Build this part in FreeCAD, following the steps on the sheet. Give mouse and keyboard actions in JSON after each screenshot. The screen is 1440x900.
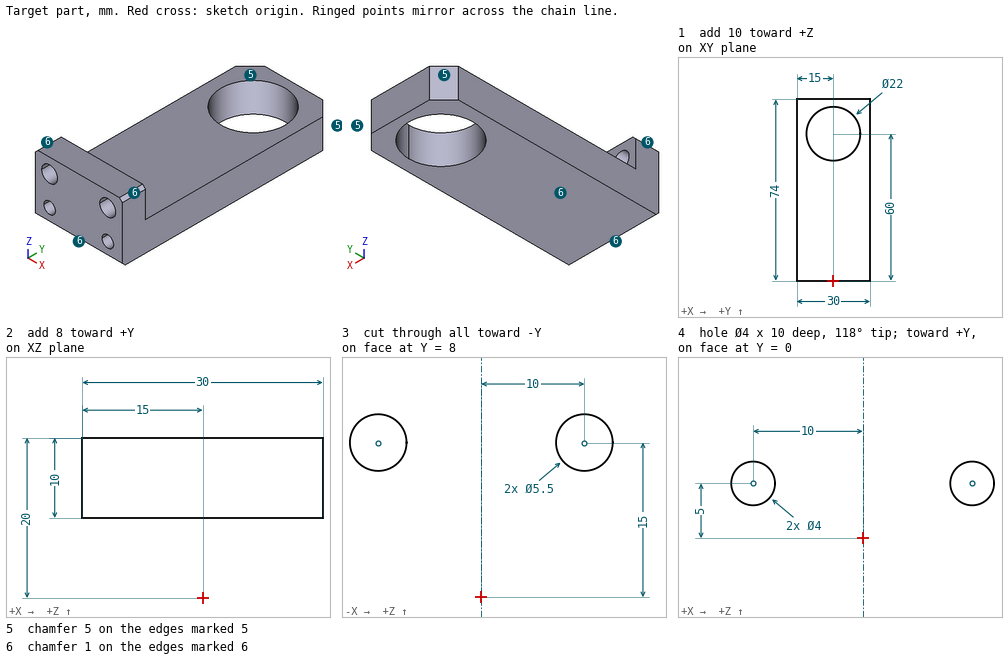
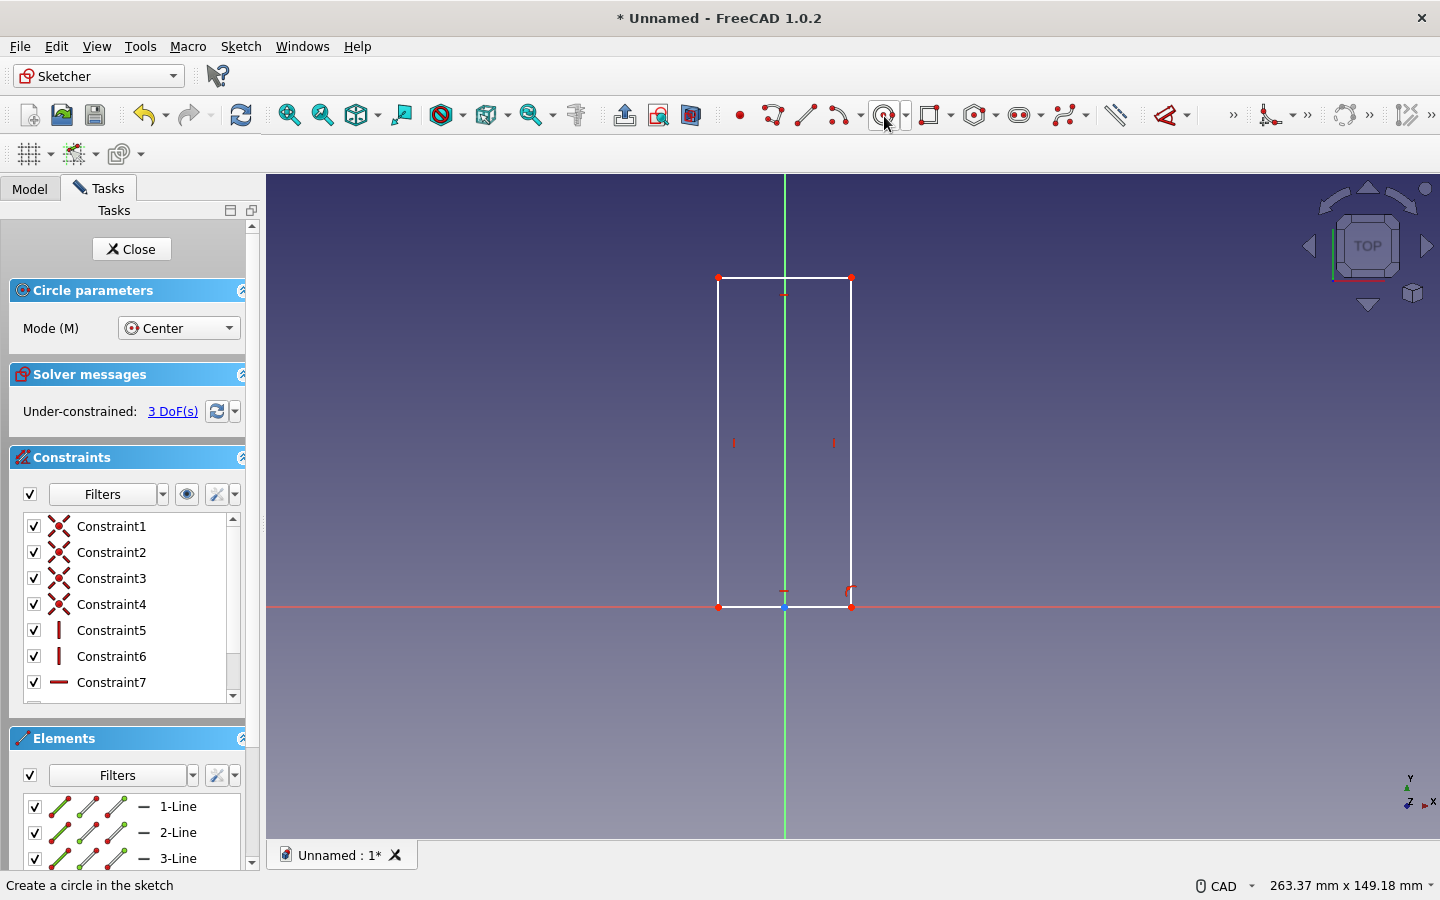
{"action": "left_click", "coordinate": [785, 340]}
{"action": "left_click", "coordinate": [819, 305]}
{"action": "key", "text": "Escape"}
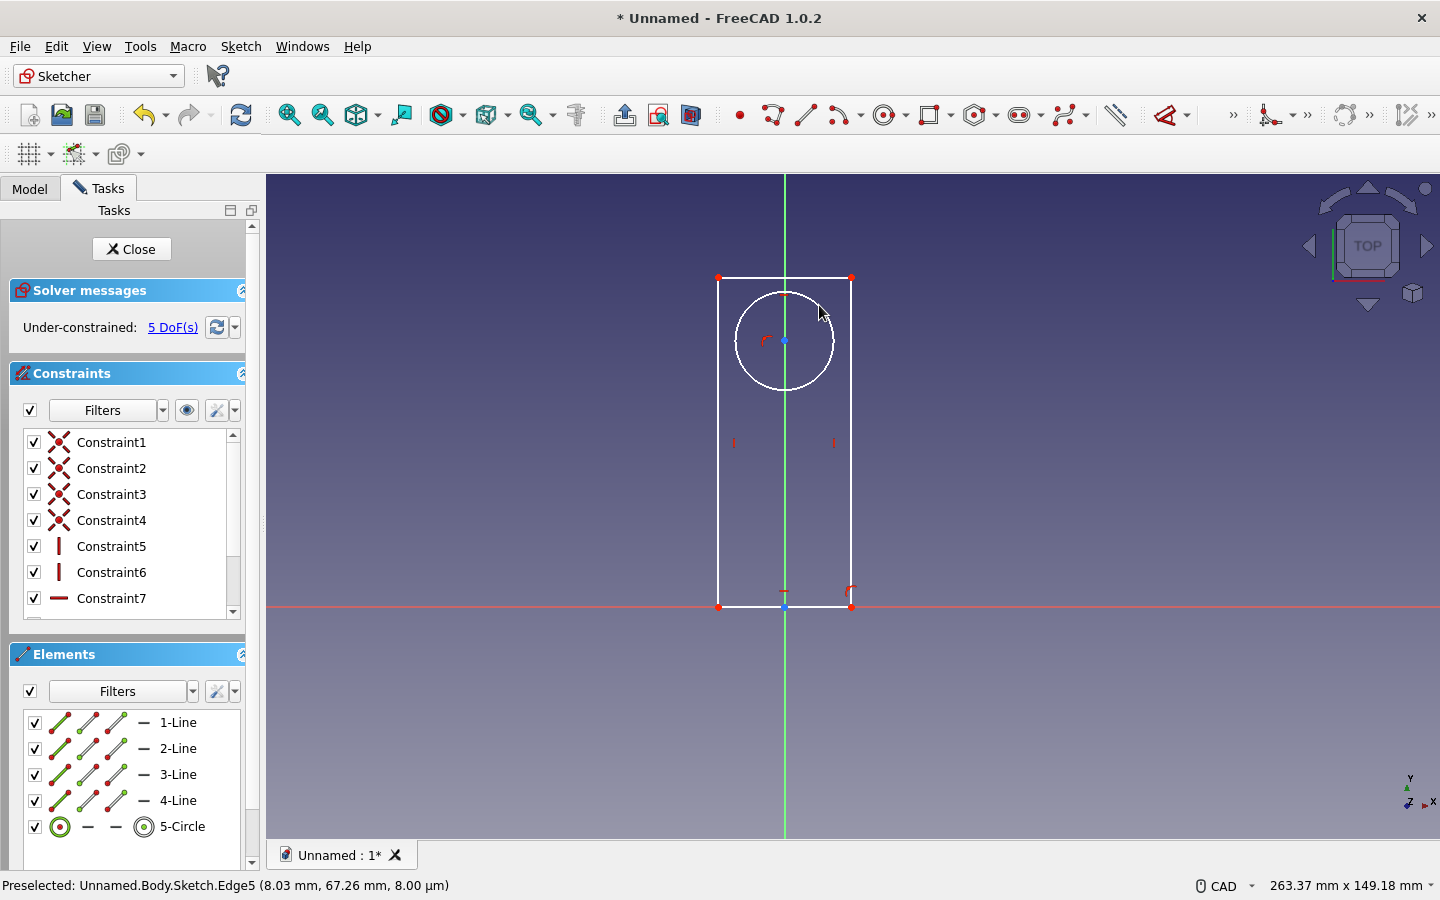
{"action": "left_click", "coordinate": [1164, 116]}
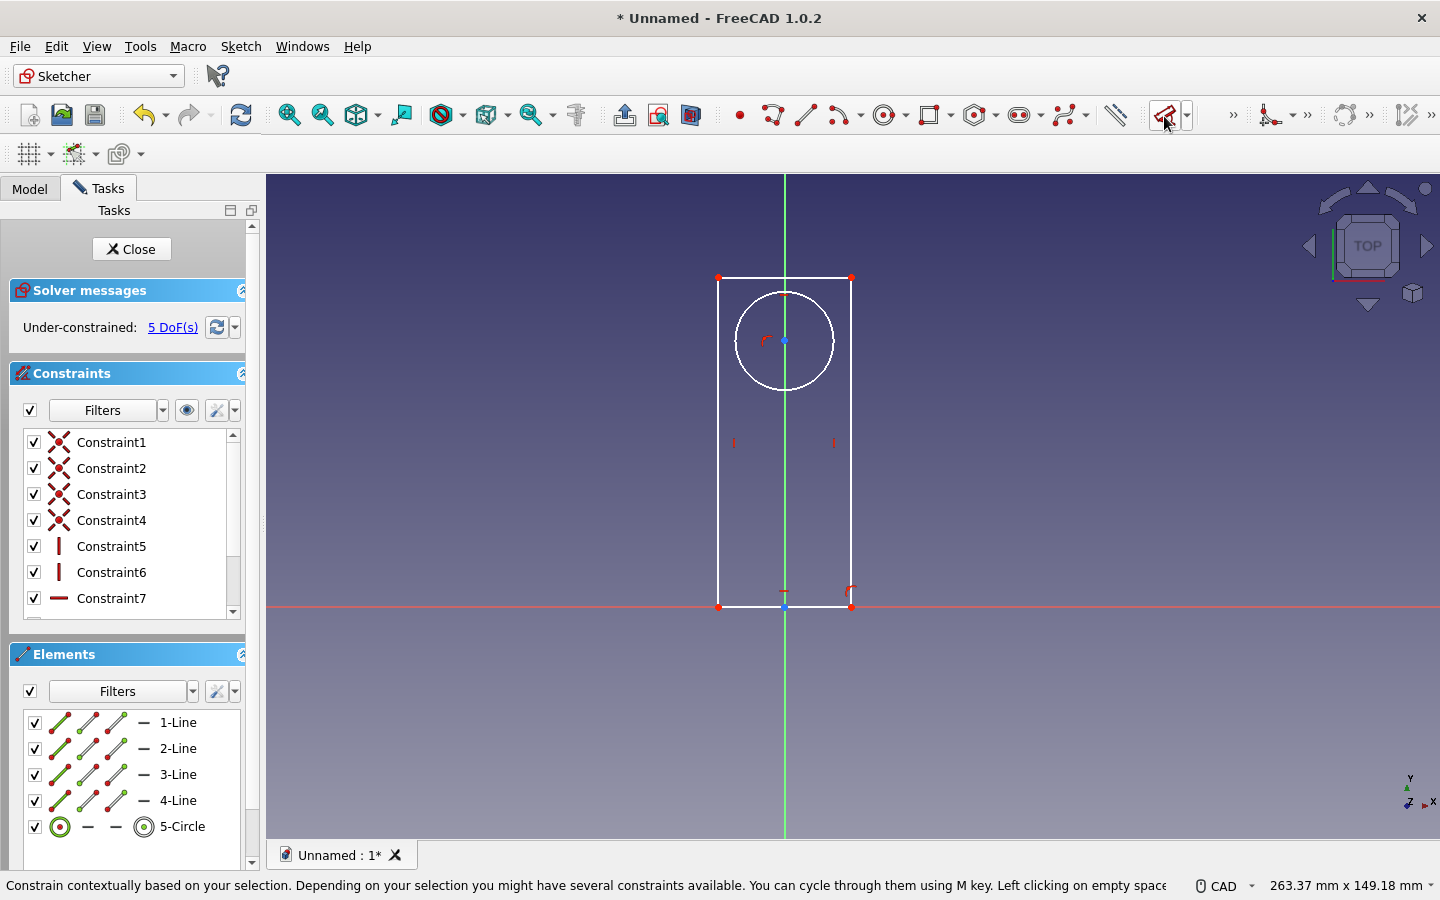
{"action": "left_click", "coordinate": [819, 306]}
{"action": "left_click", "coordinate": [807, 263]}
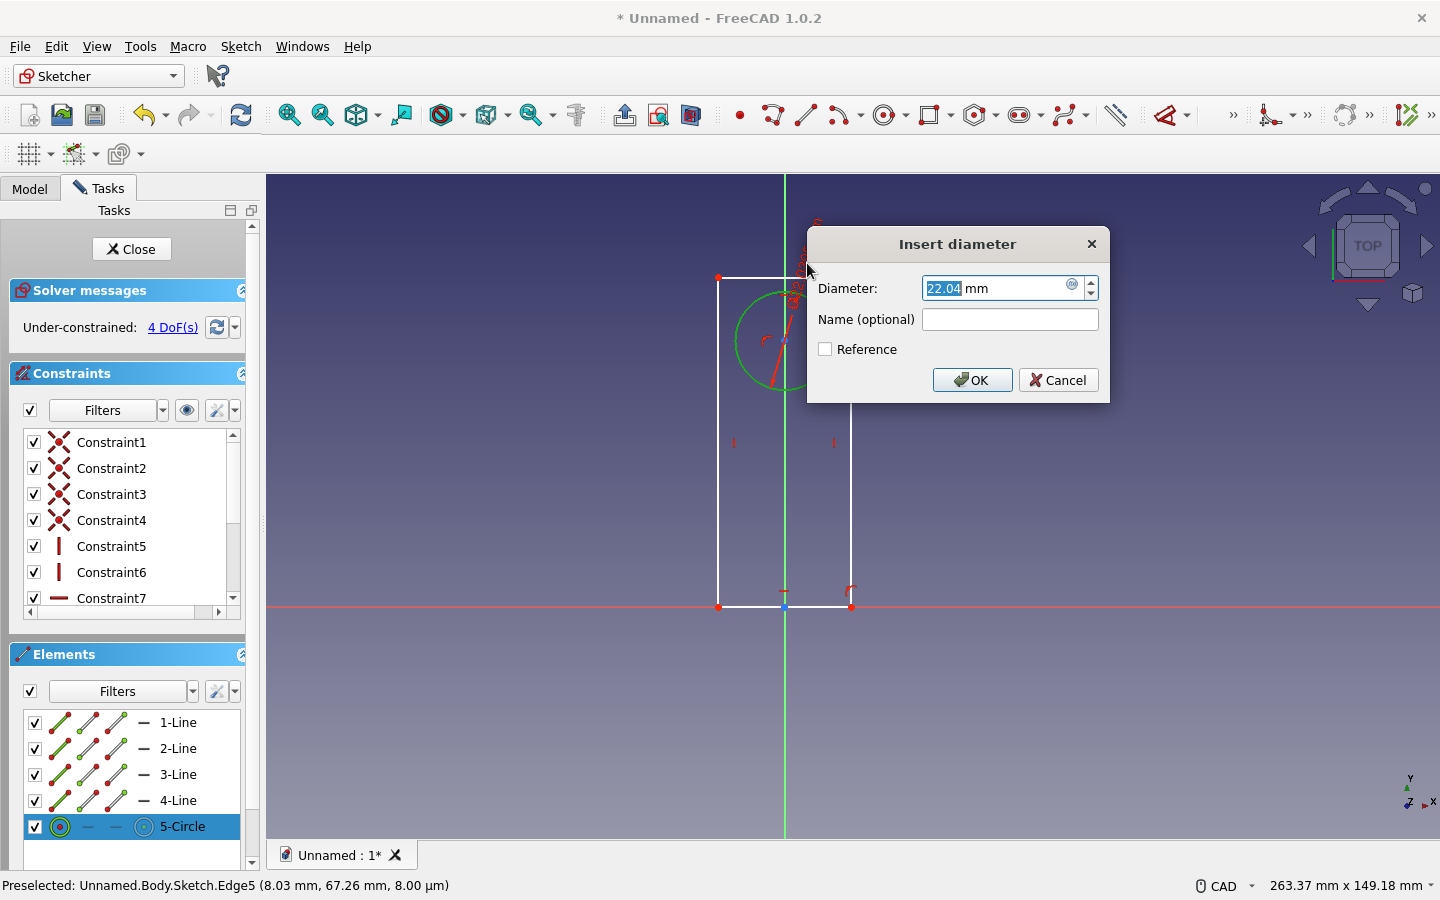
{"action": "type", "text": "22"}
{"action": "key", "text": "Return"}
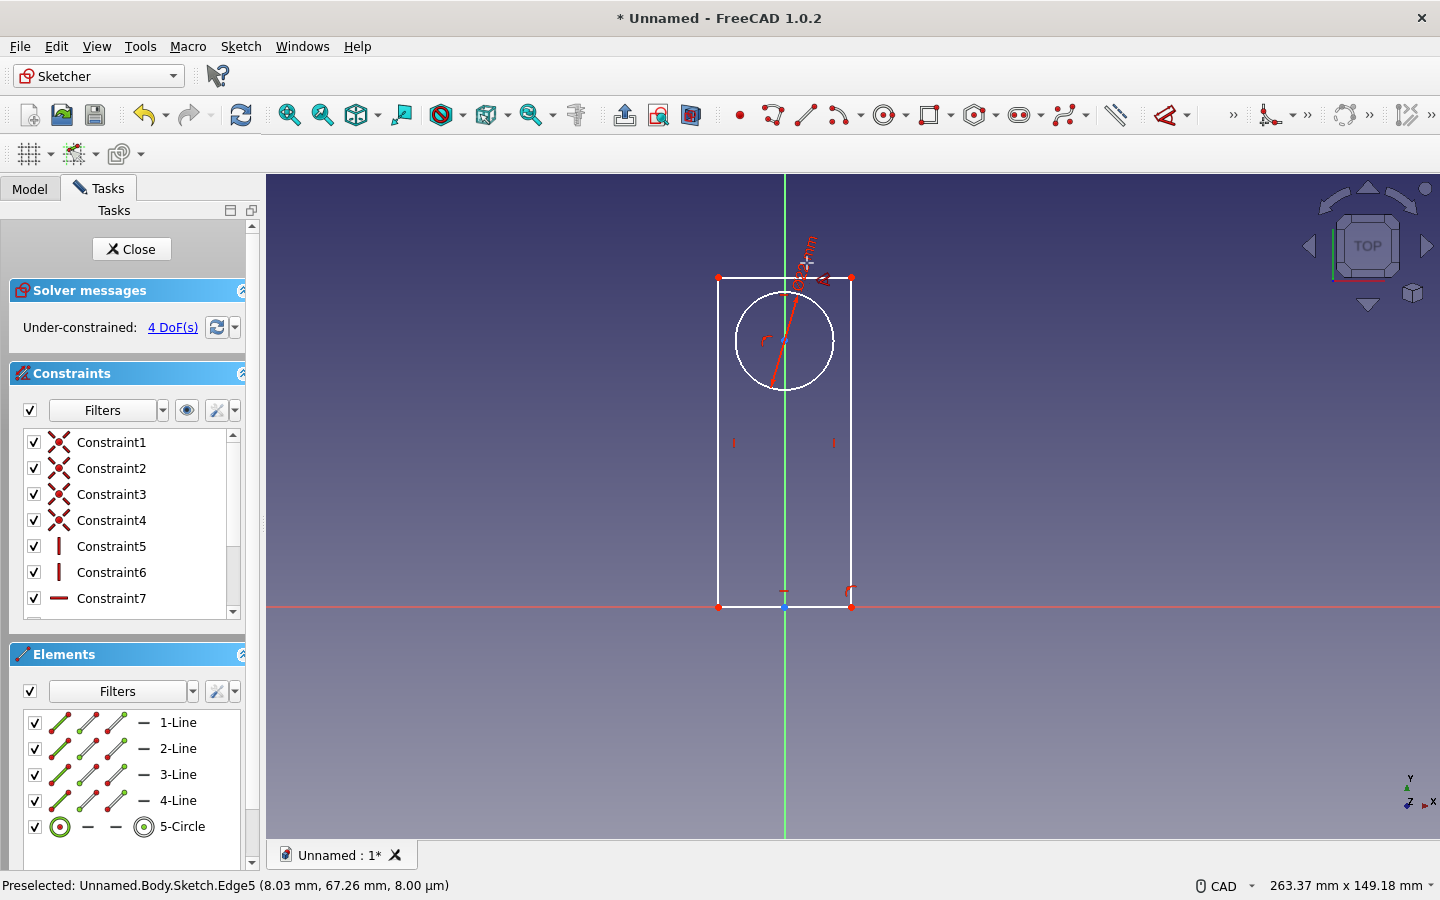
{"action": "left_click", "coordinate": [718, 377]}
{"action": "left_click", "coordinate": [684, 443]}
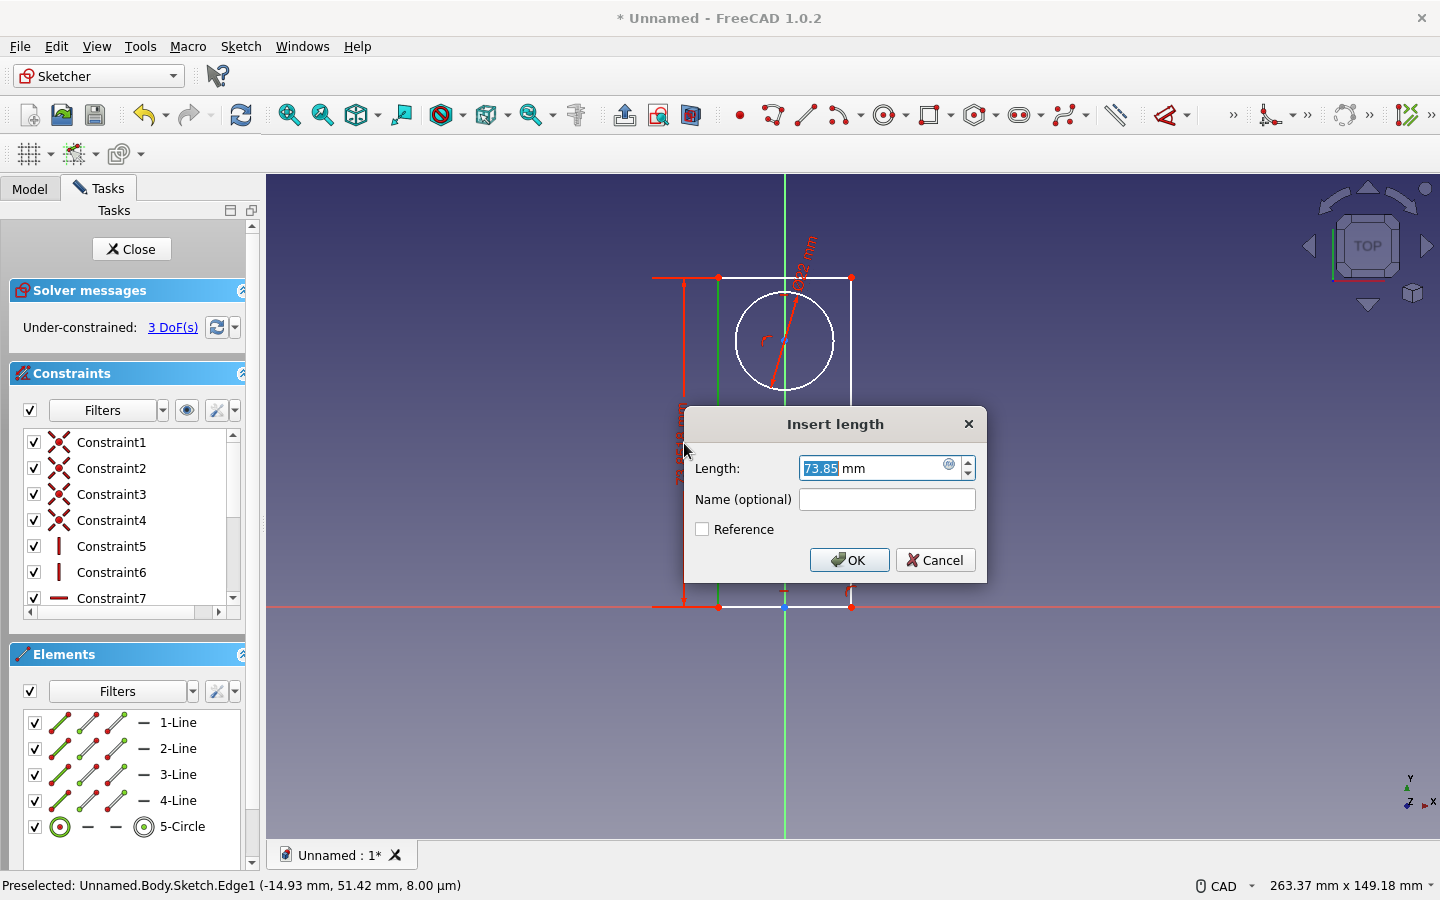
{"action": "type", "text": "74"}
{"action": "key", "text": "Return"}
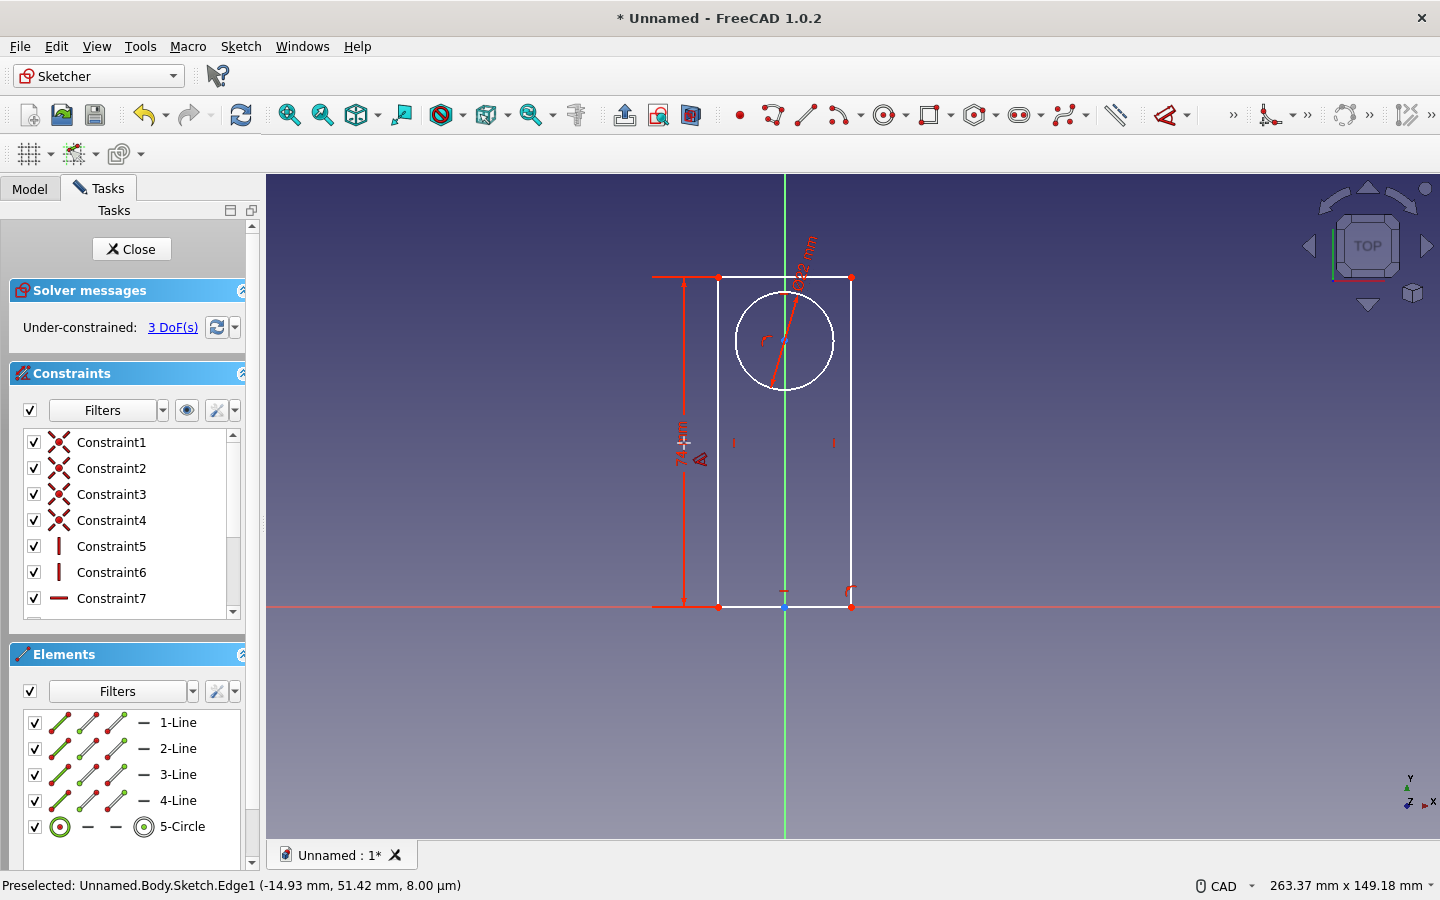
{"action": "left_click", "coordinate": [758, 607]}
{"action": "left_click", "coordinate": [754, 641]}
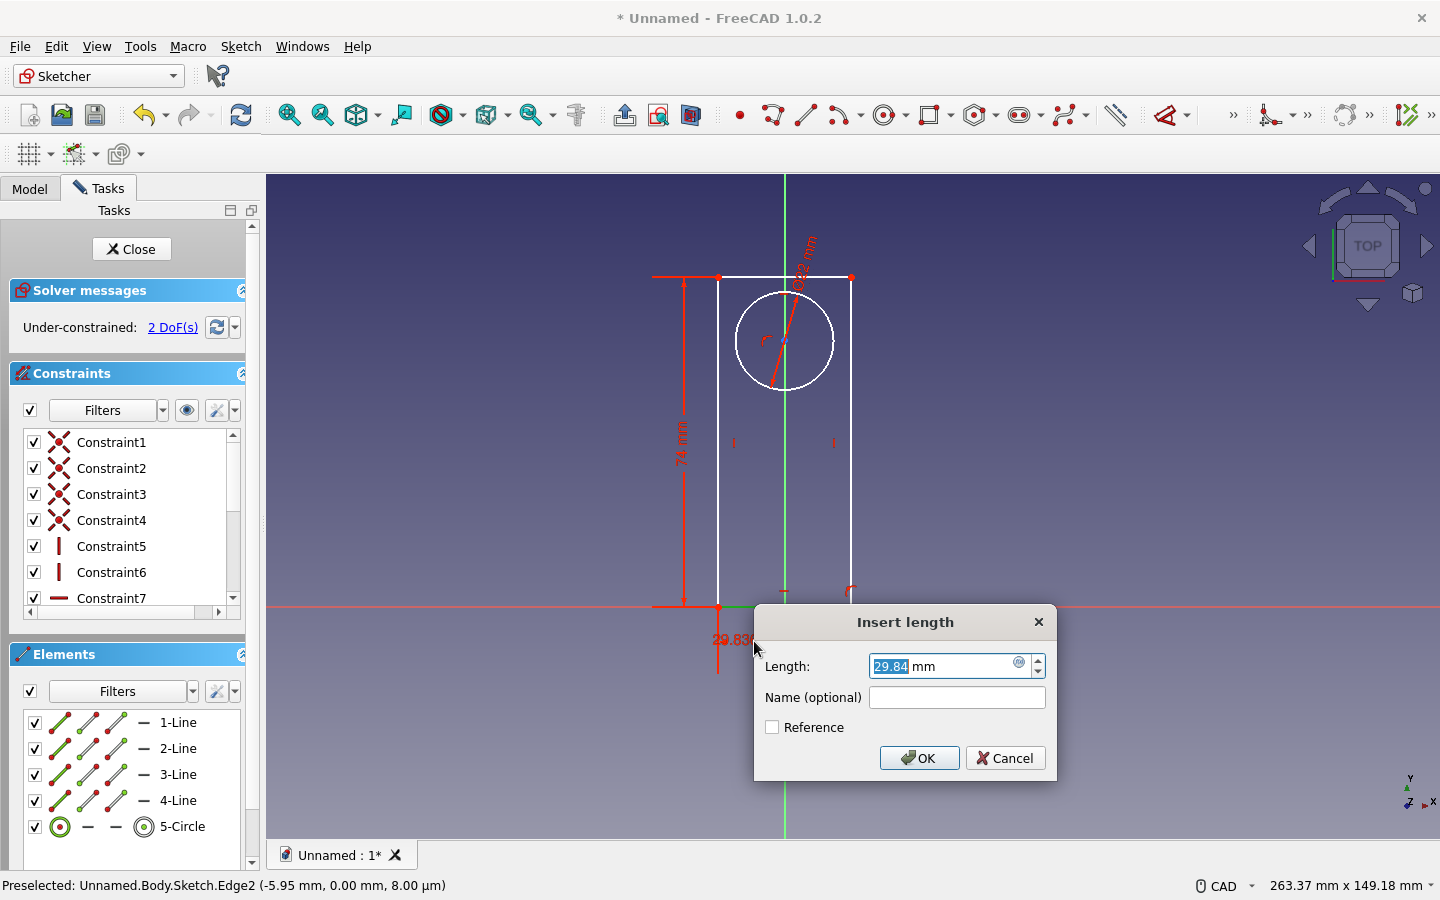
{"action": "type", "text": "30"}
{"action": "key", "text": "Return"}